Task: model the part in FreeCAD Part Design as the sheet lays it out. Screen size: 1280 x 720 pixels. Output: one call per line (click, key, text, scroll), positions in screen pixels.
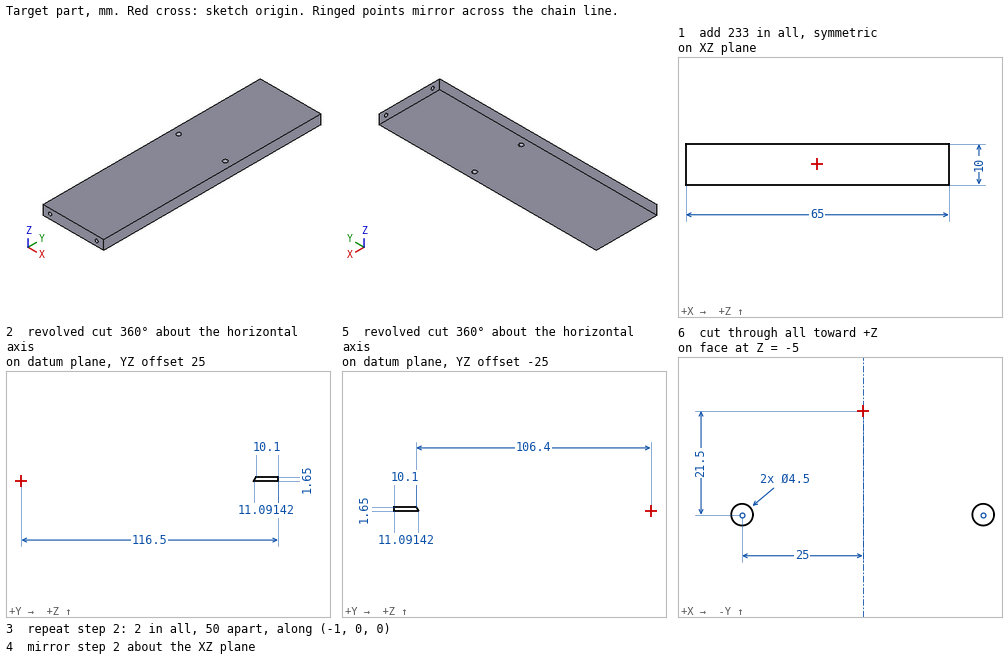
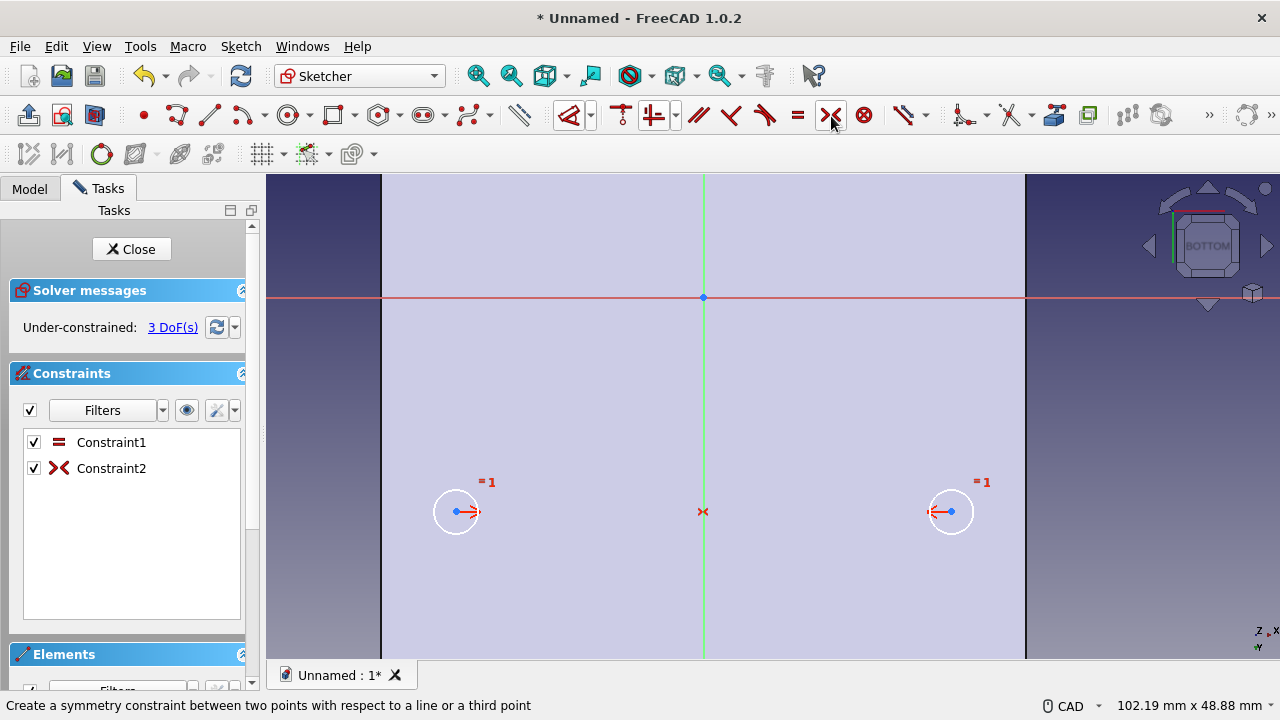
click(471, 496)
click(493, 473)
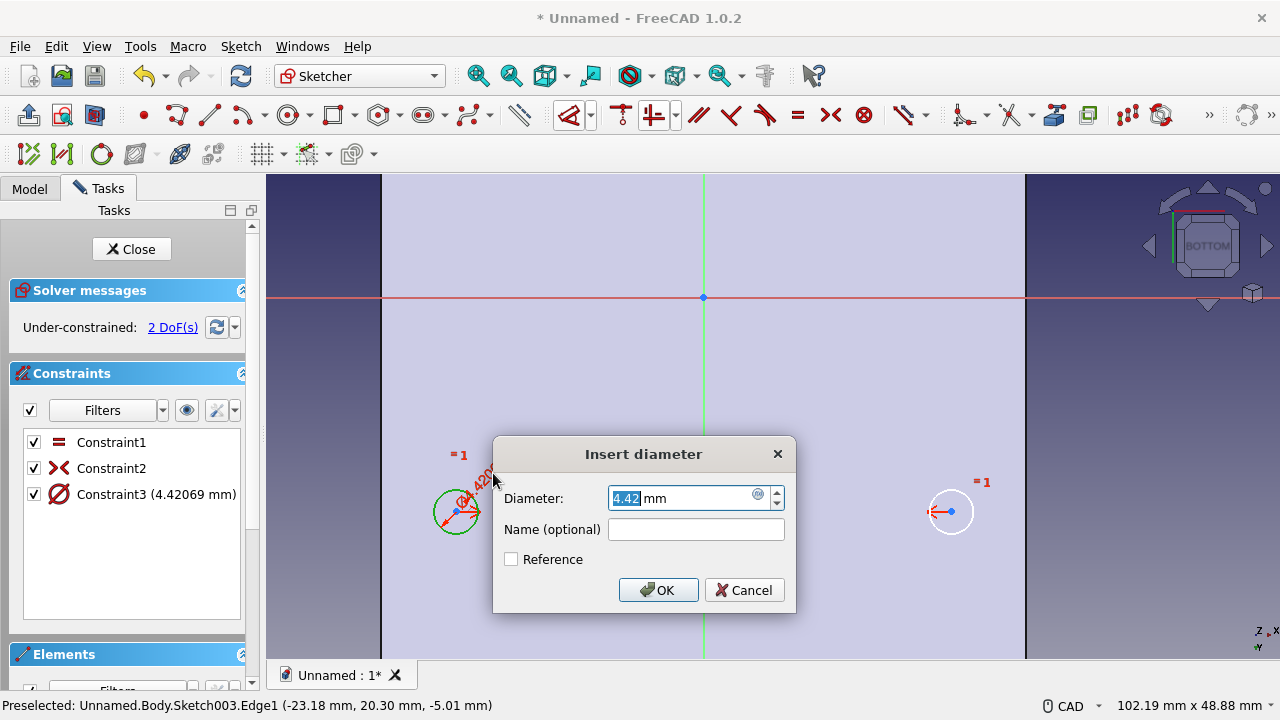
text(4.5)
key(Return)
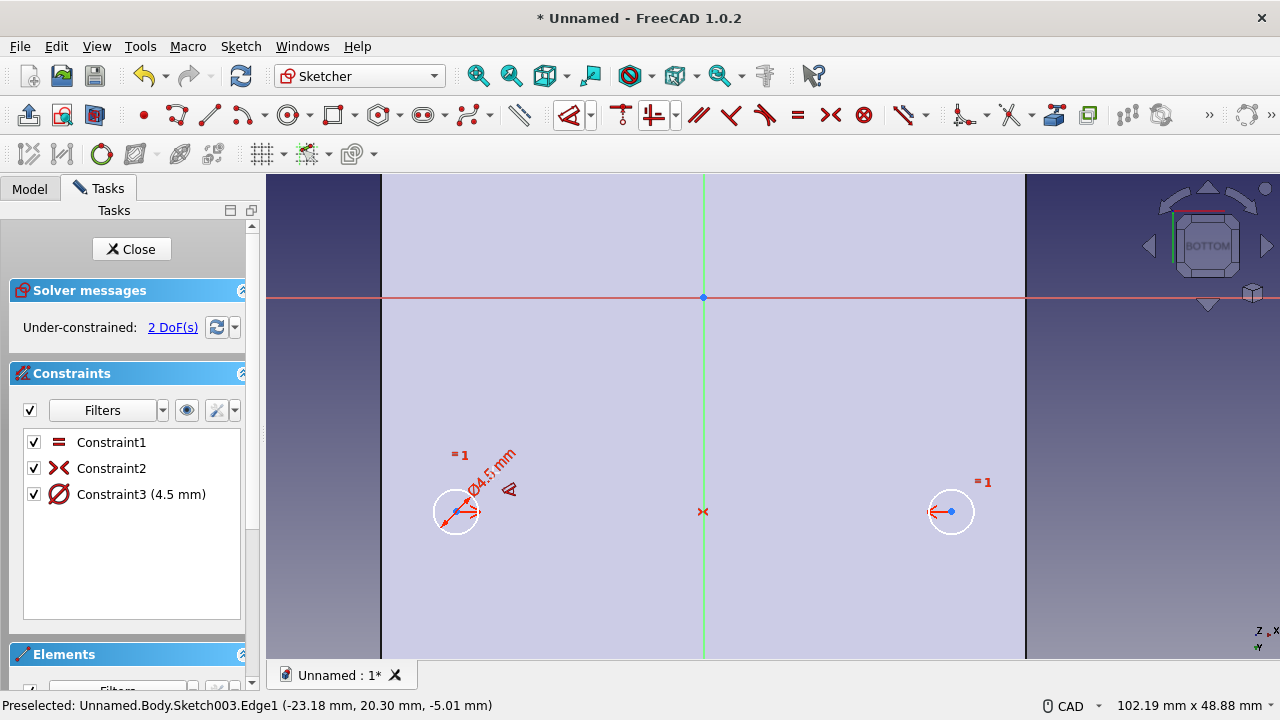
click(456, 512)
click(580, 264)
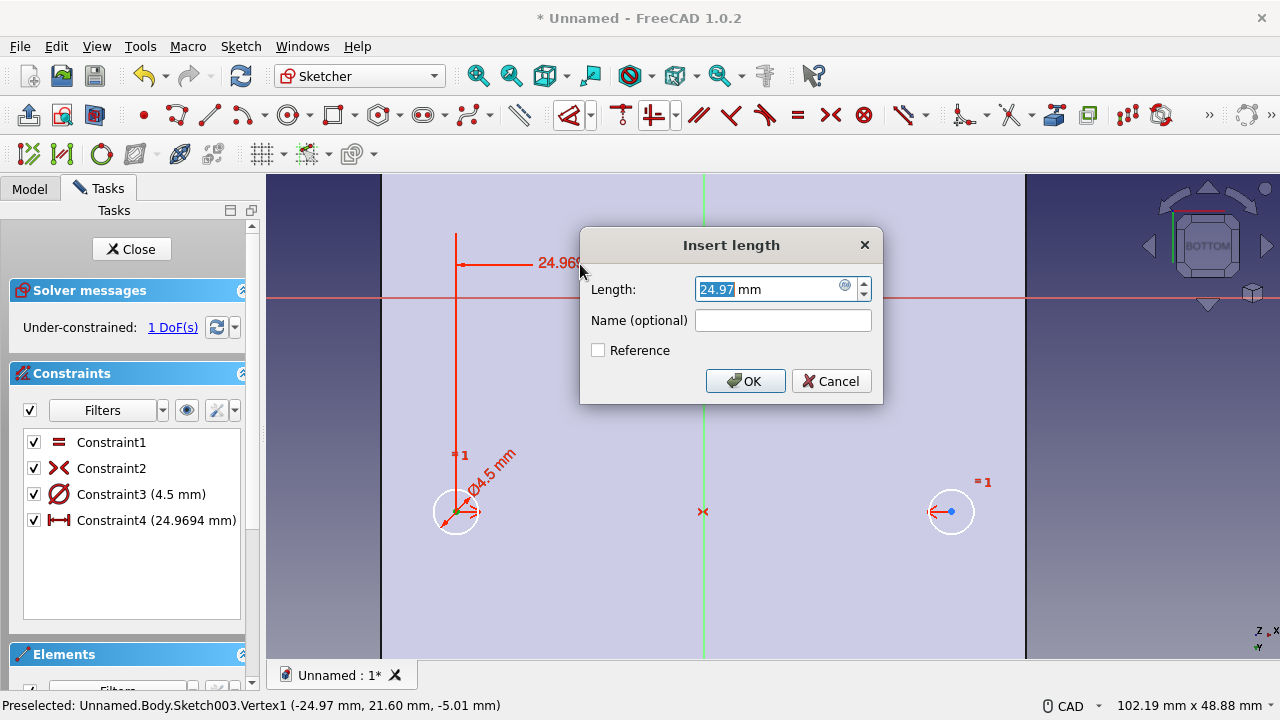
text(25)
key(Return)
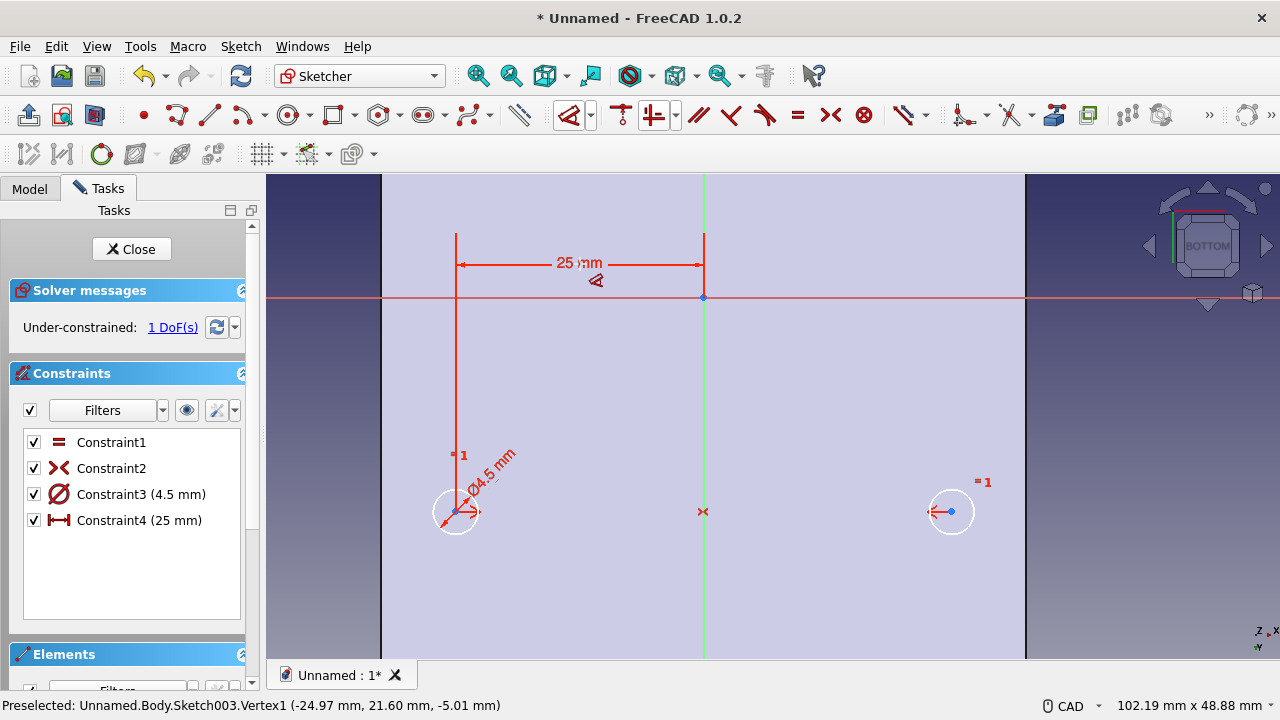
click(456, 512)
click(422, 405)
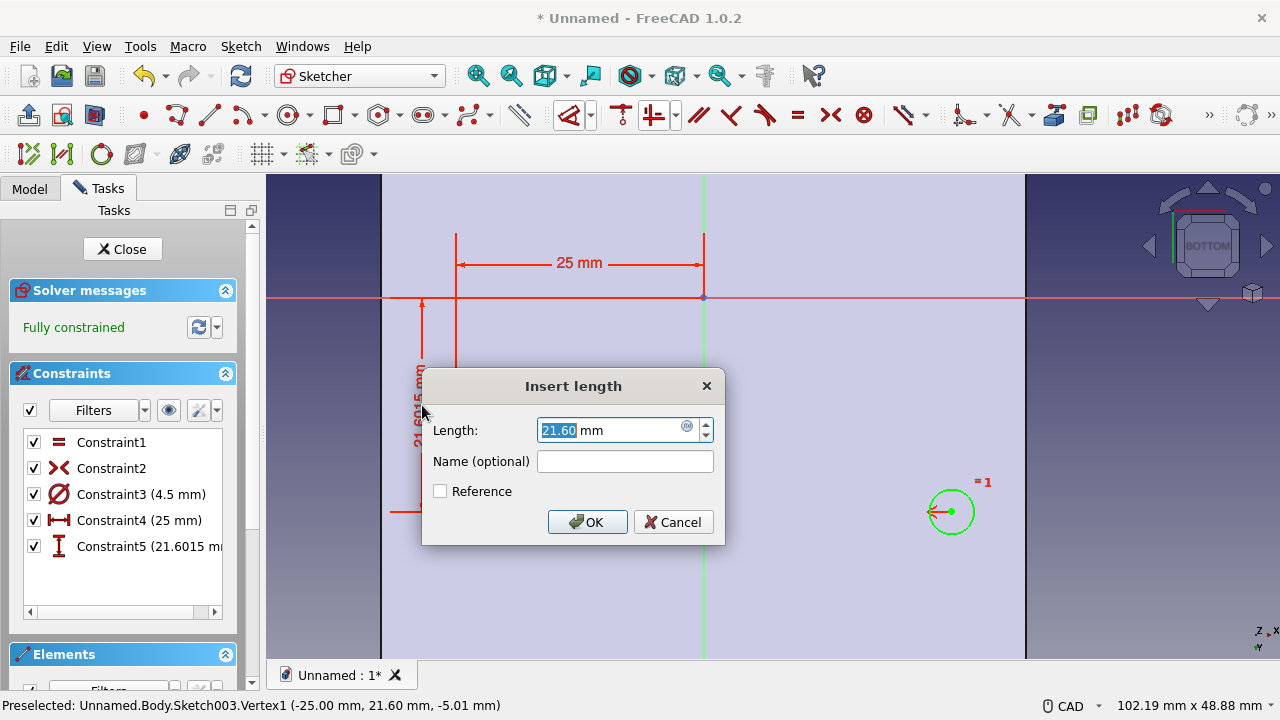
text(21.5)
key(Return)
key(Escape)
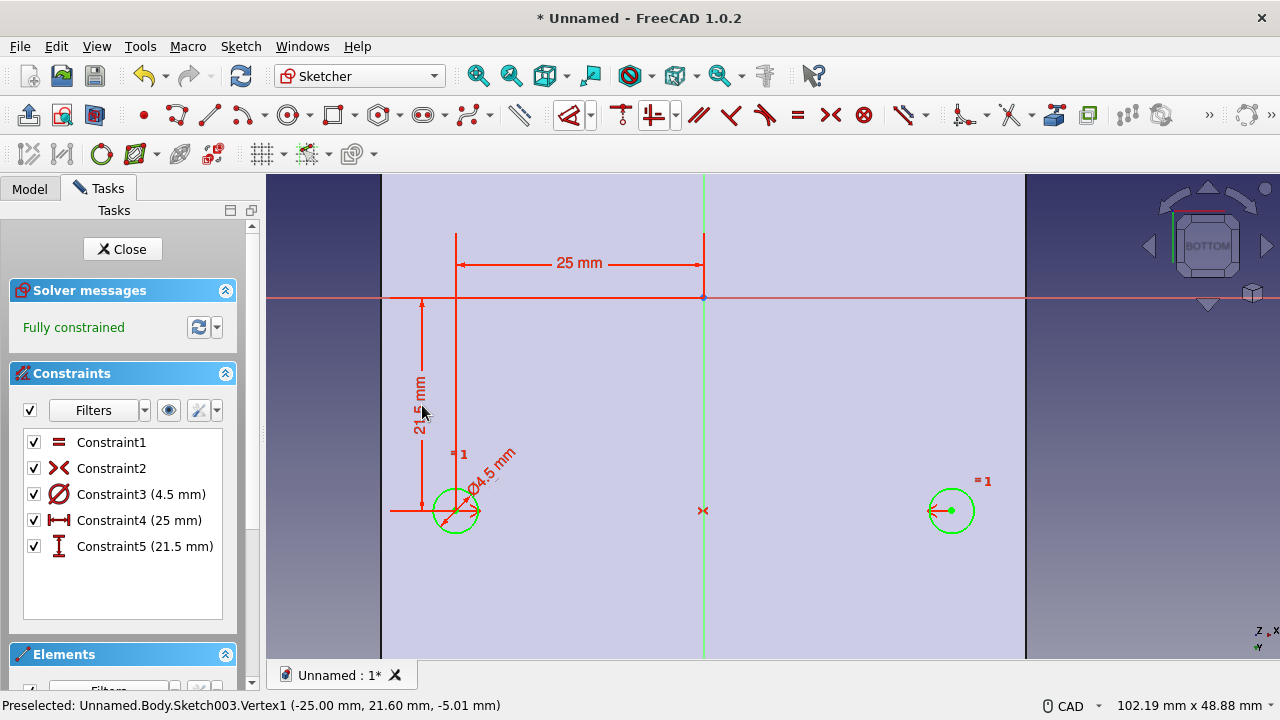
click(123, 249)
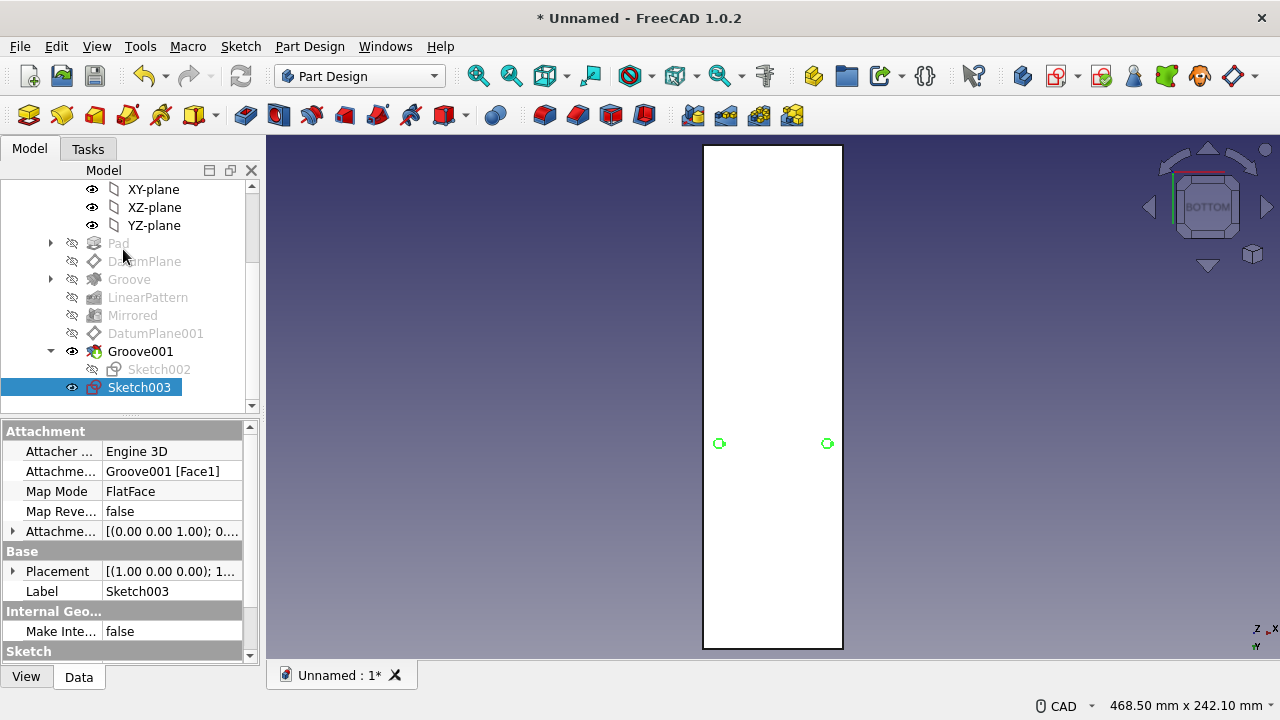
click(246, 116)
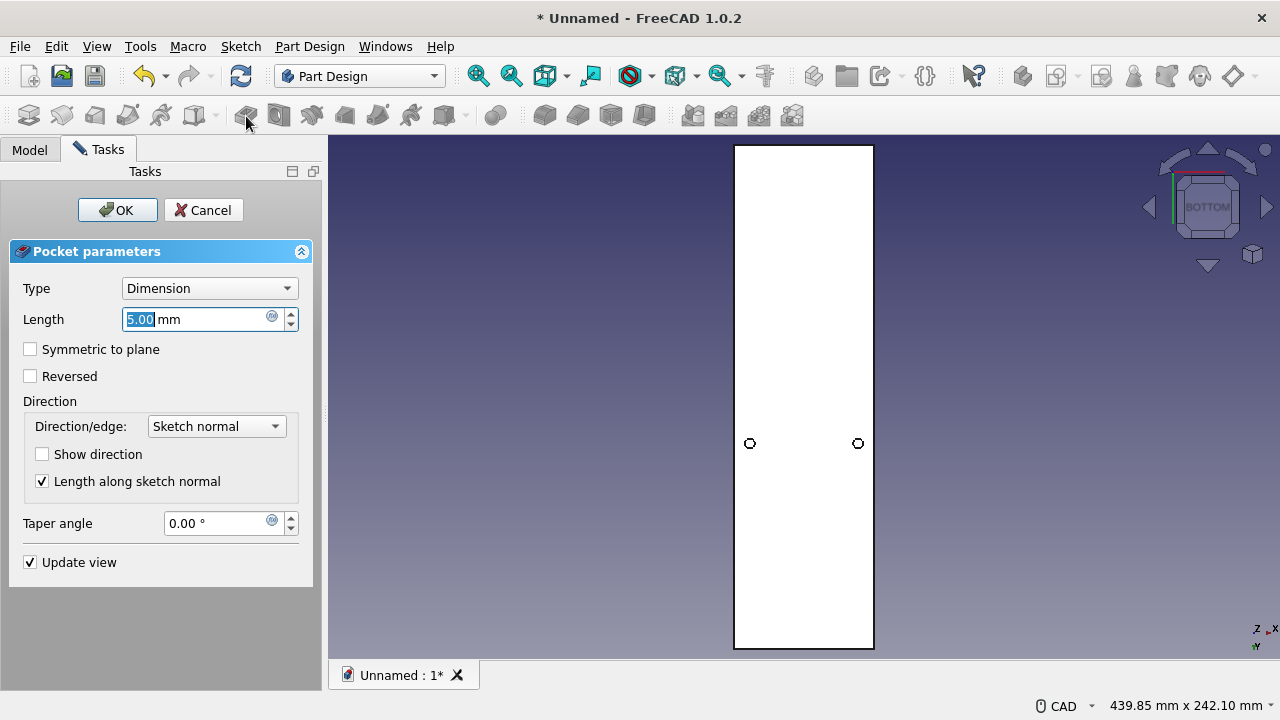
click(210, 288)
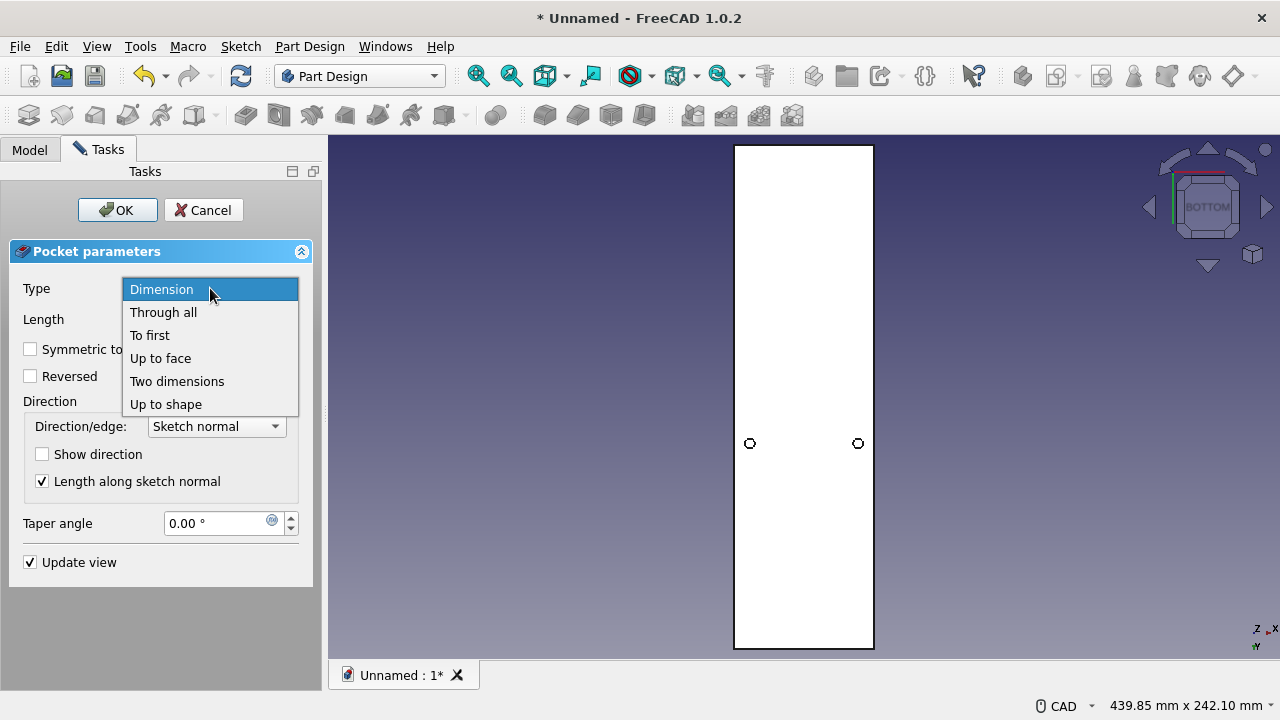
click(208, 312)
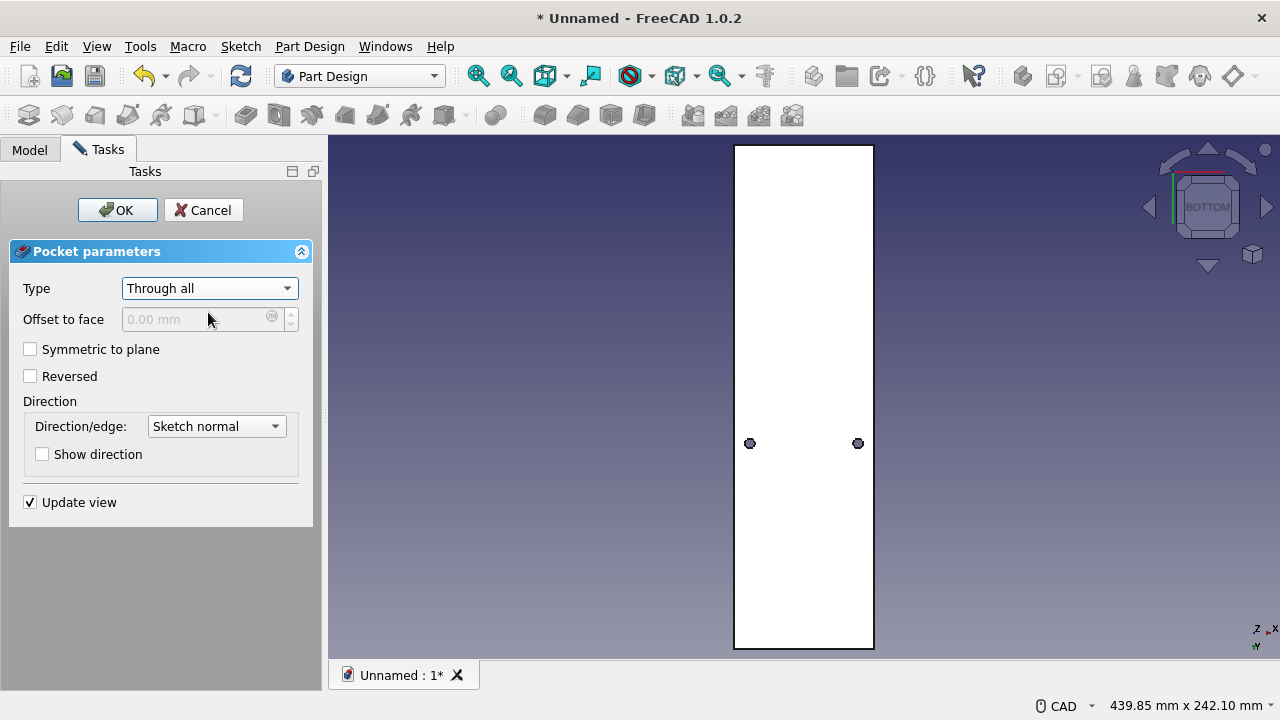
click(118, 210)